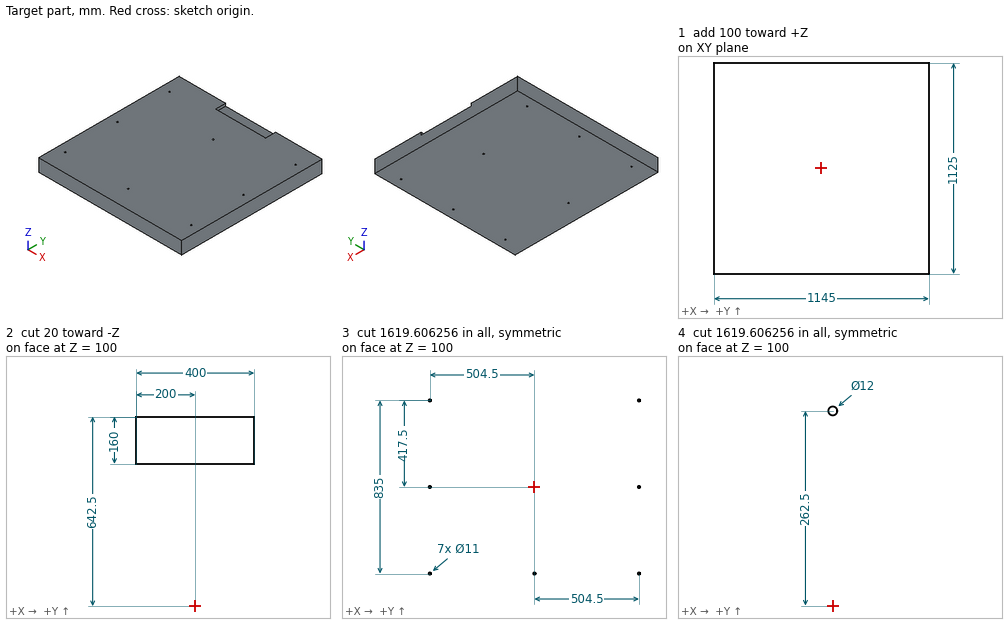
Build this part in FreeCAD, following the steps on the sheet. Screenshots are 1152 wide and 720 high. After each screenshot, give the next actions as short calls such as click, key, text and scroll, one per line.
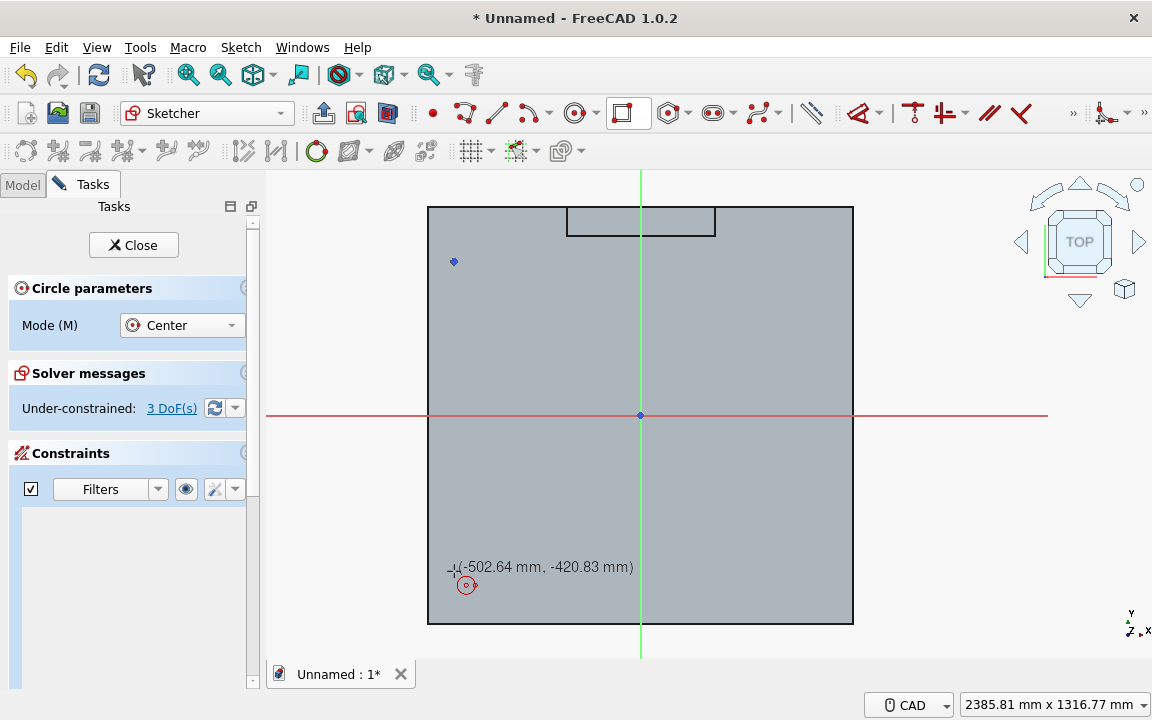
click(454, 571)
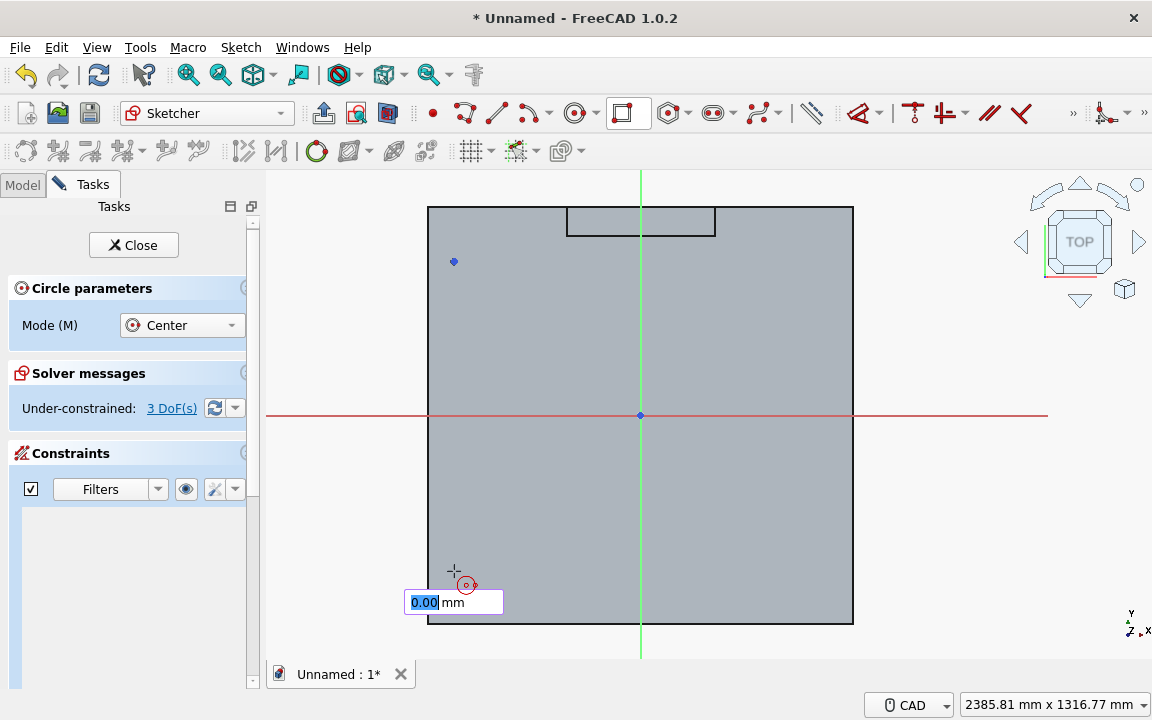
scroll(455, 569, up, 11)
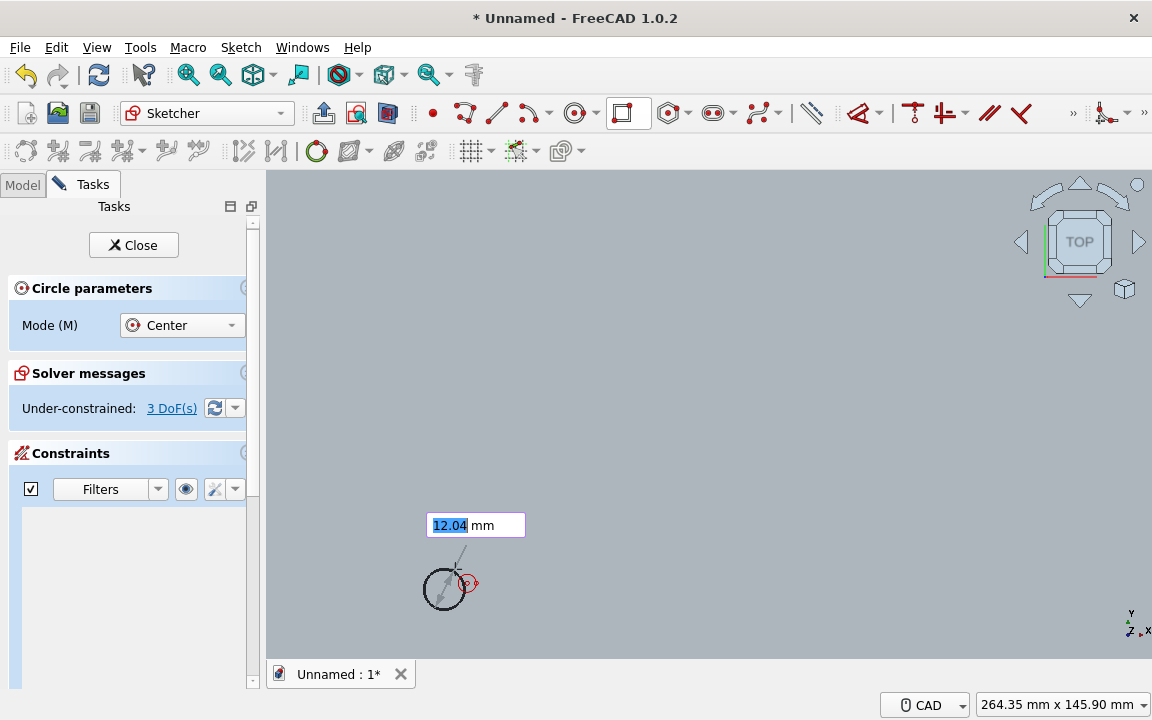
click(453, 564)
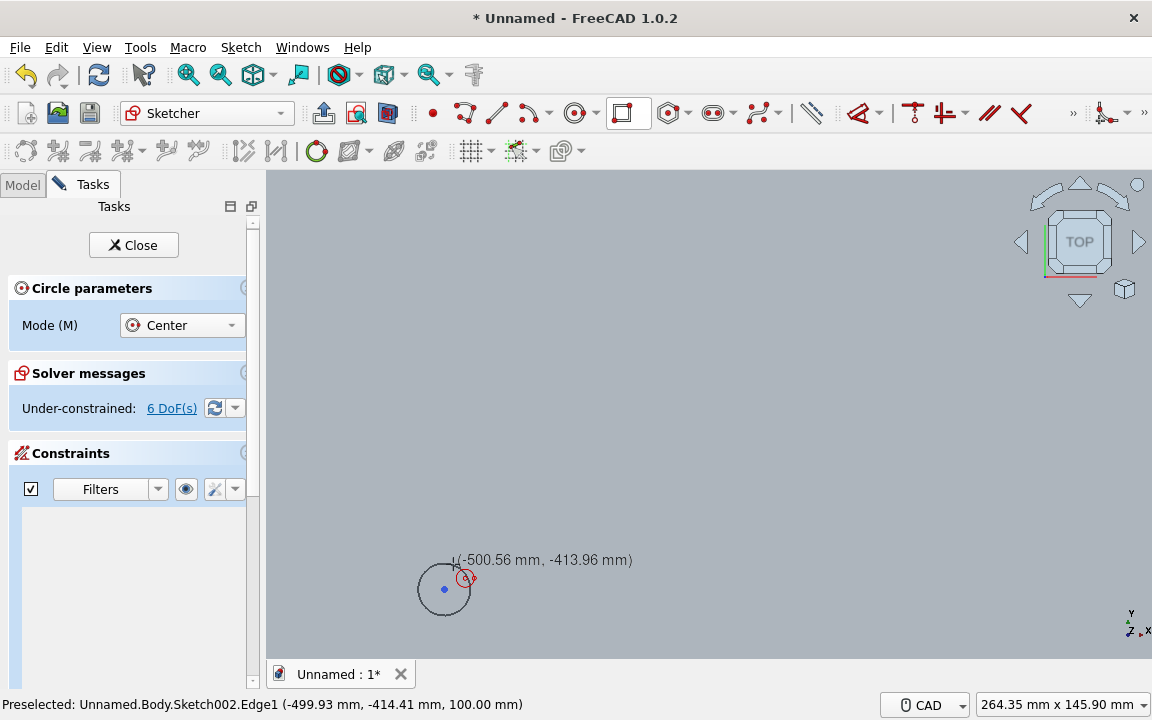
scroll(455, 569, down, 11)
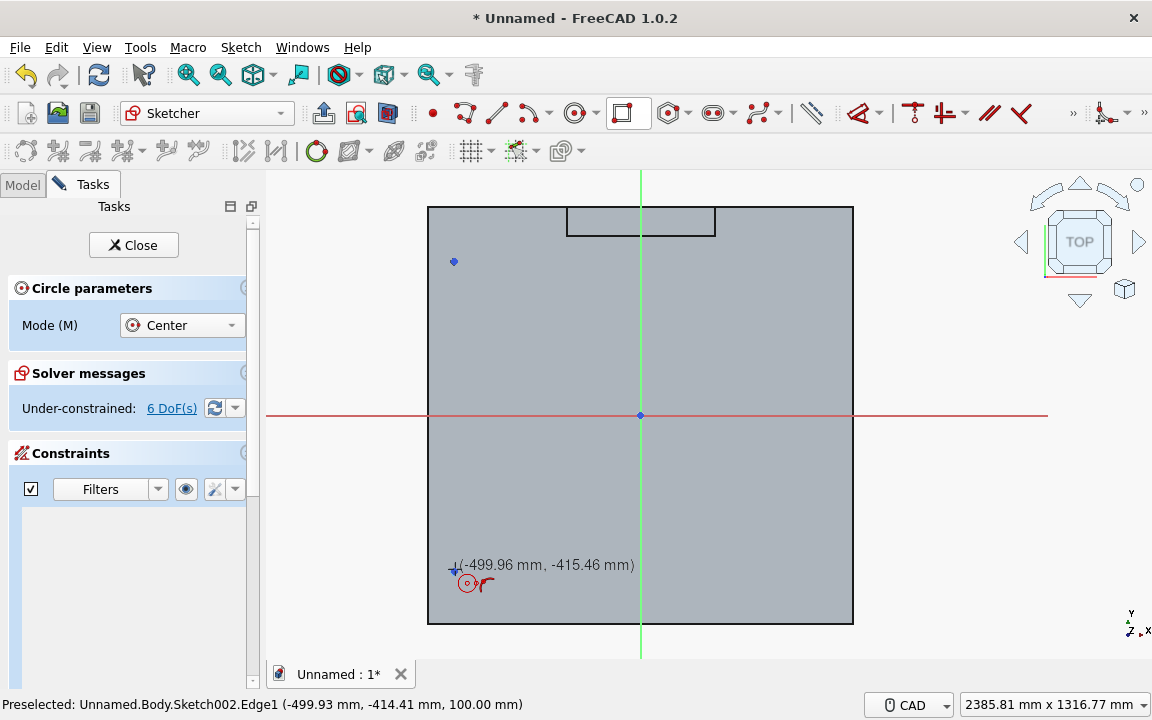
scroll(828, 571, up, 13)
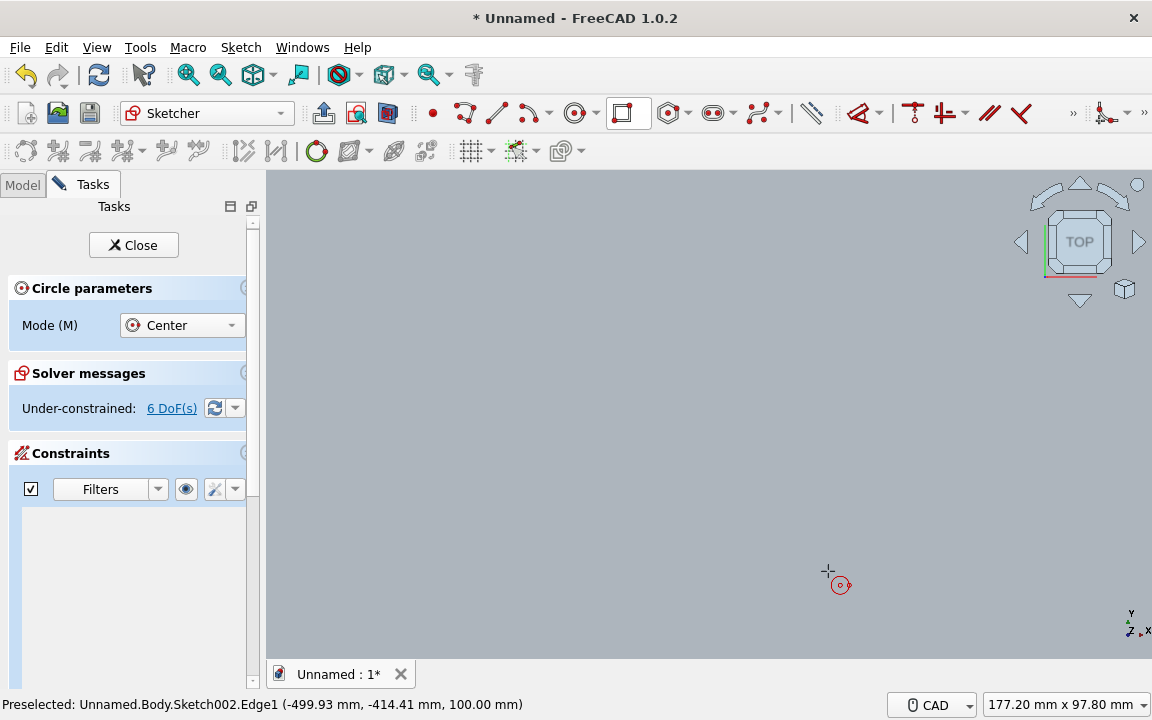
scroll(828, 571, down, 13)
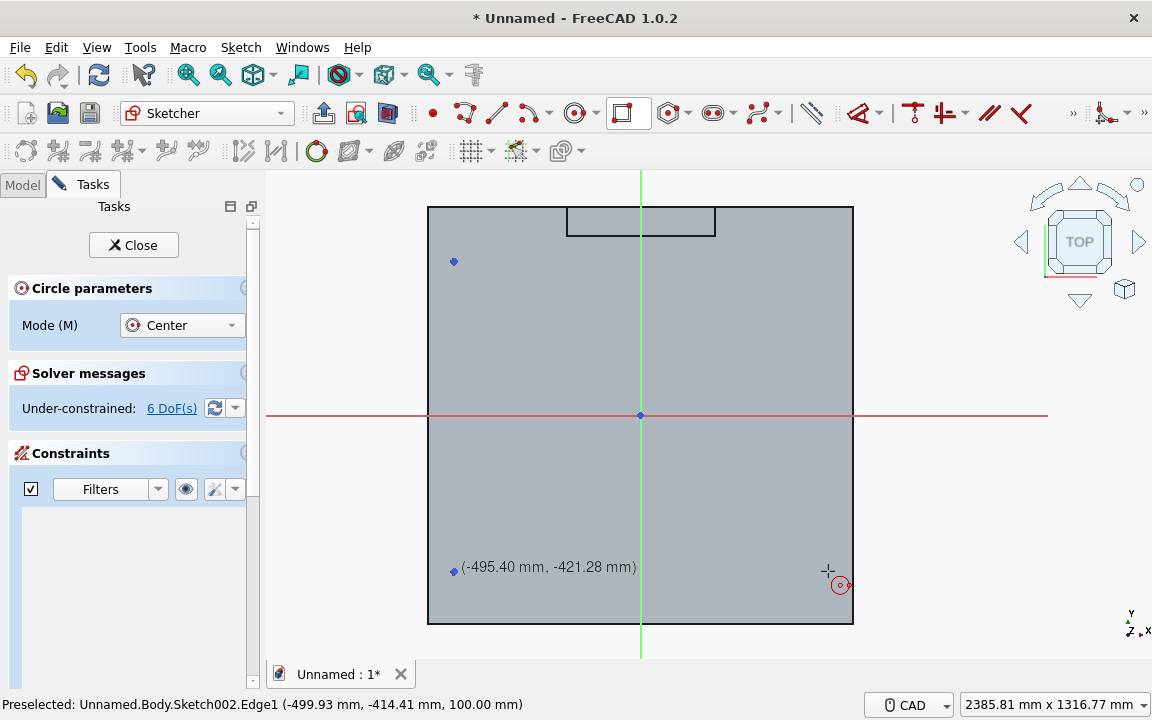
click(828, 571)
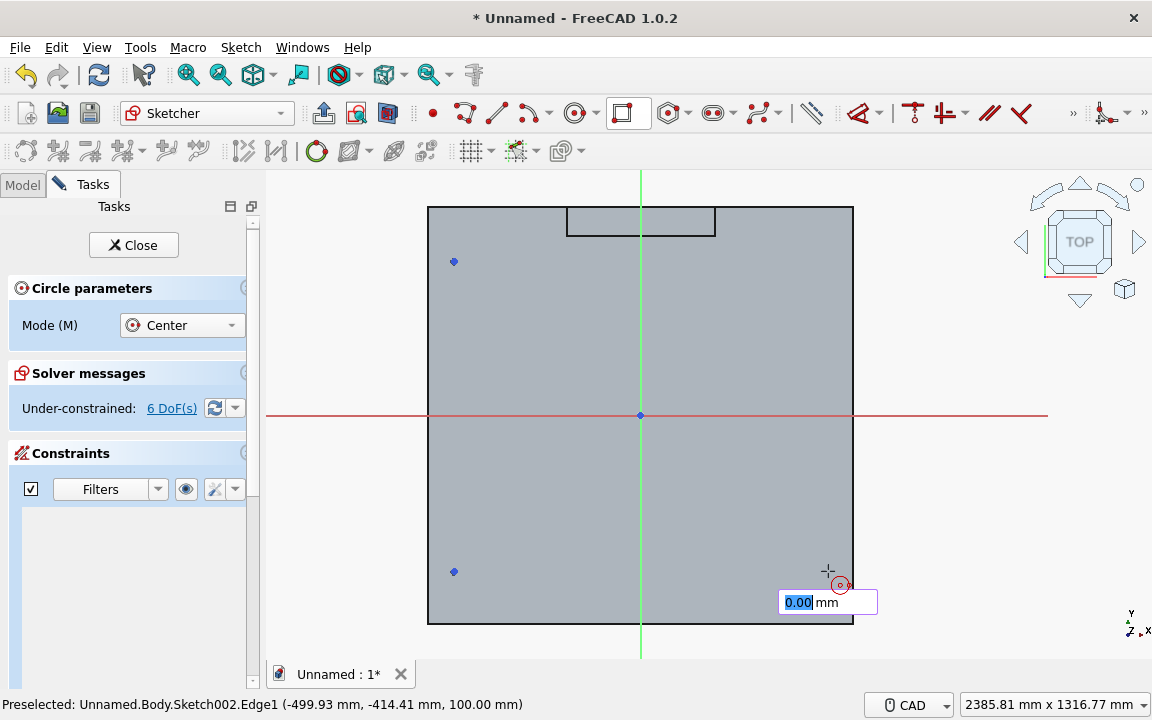
scroll(830, 569, up, 11)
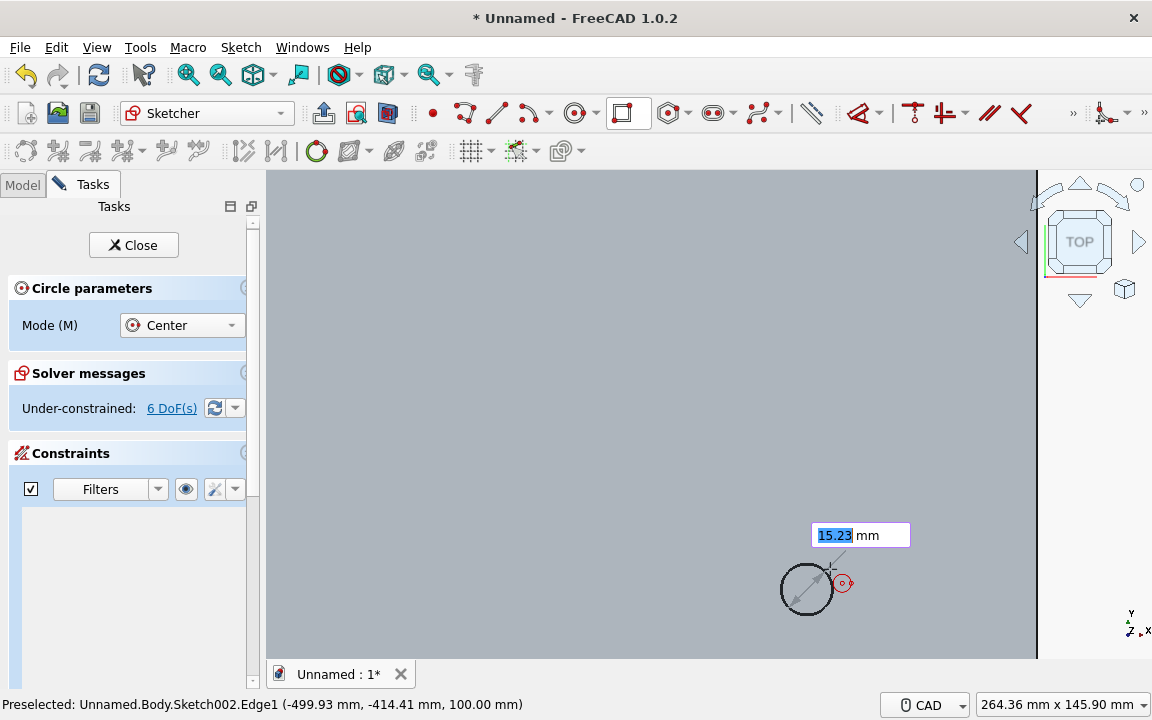
click(822, 564)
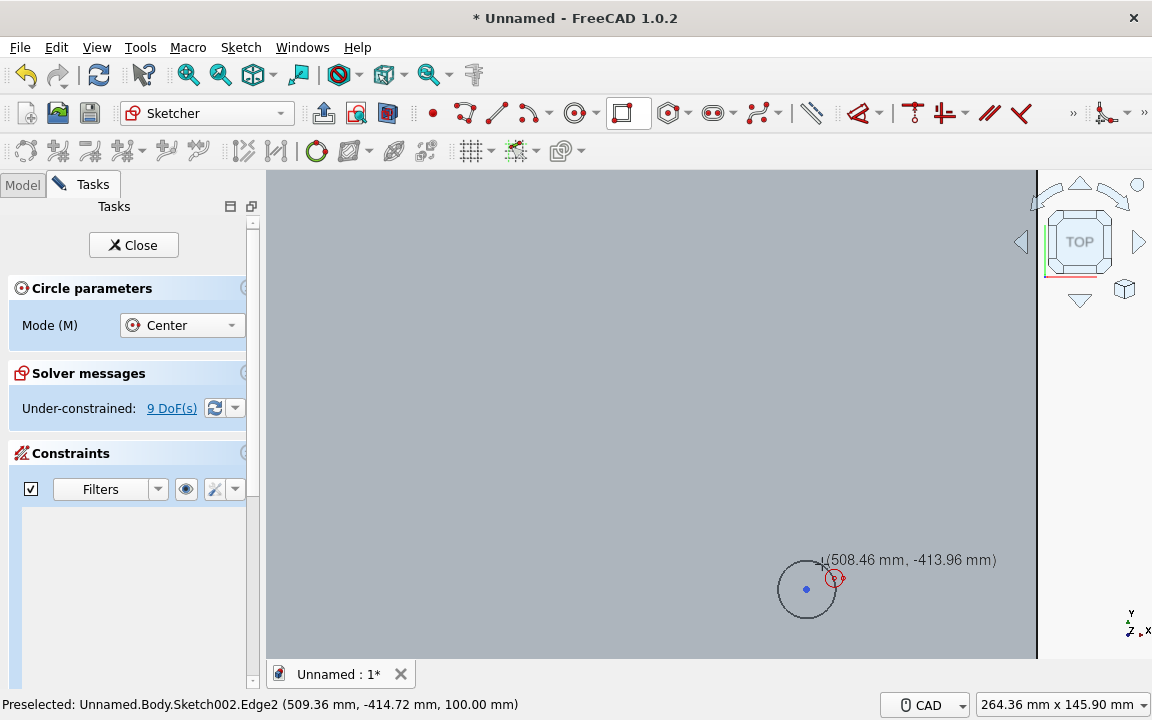
scroll(830, 569, down, 11)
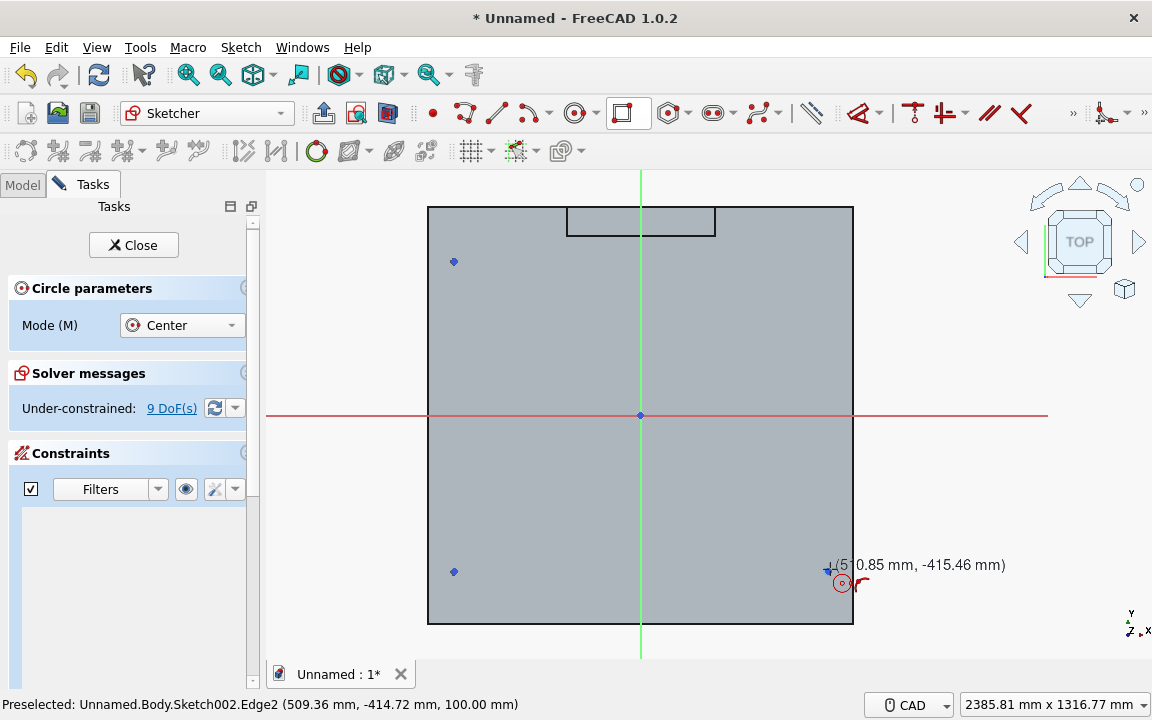
scroll(828, 261, up, 13)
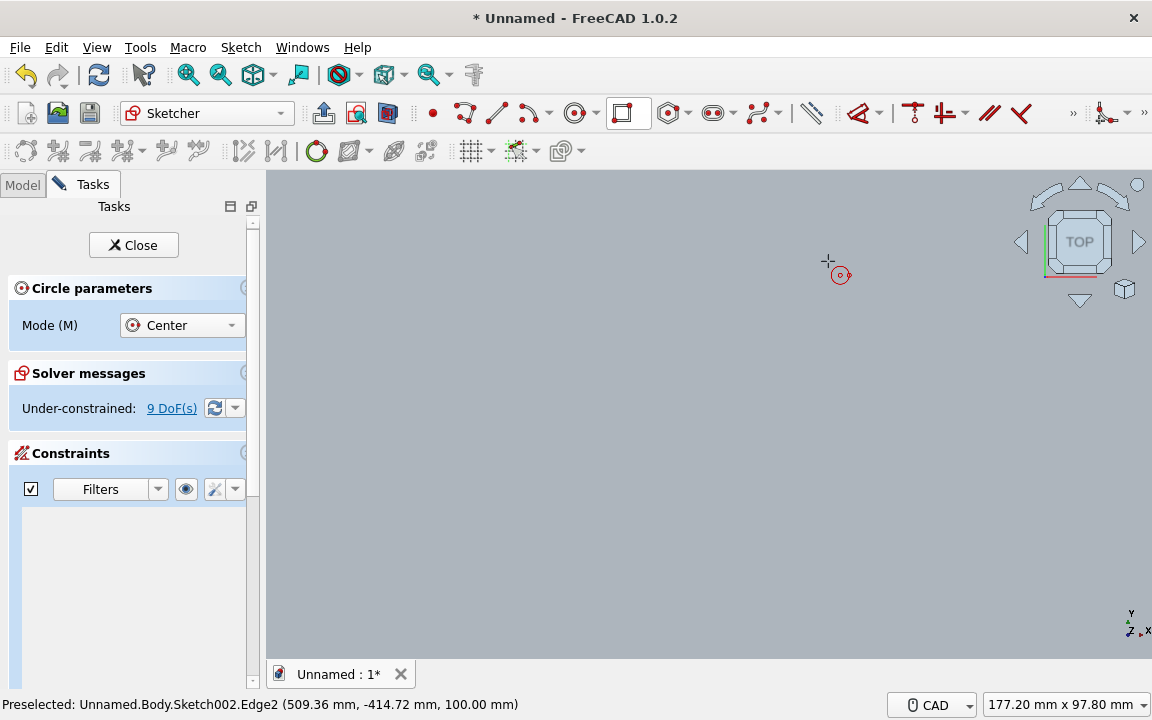
scroll(828, 260, down, 13)